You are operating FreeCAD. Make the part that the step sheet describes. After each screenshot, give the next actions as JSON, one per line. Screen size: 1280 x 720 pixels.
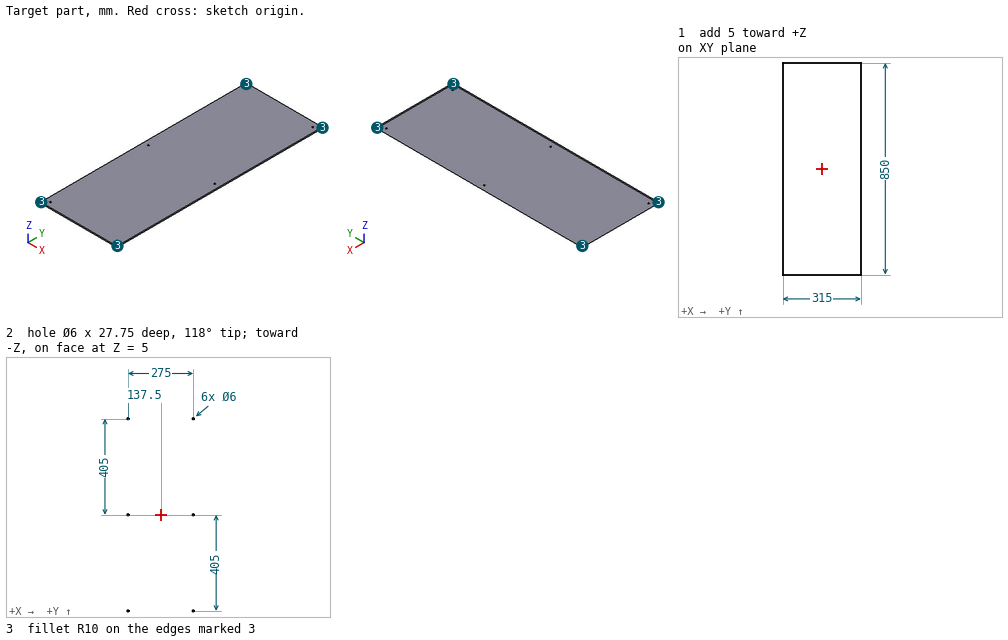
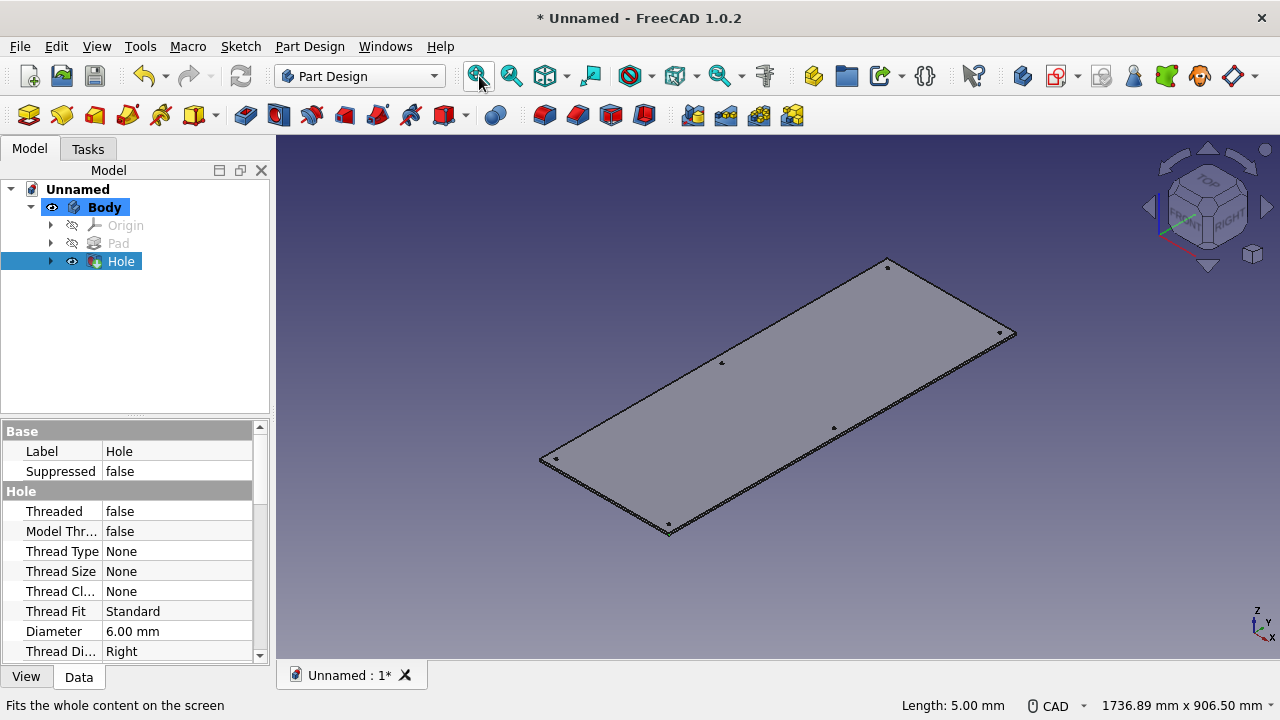
{"action": "scroll", "coordinate": [540, 459], "scroll_direction": "up", "scroll_amount": 14}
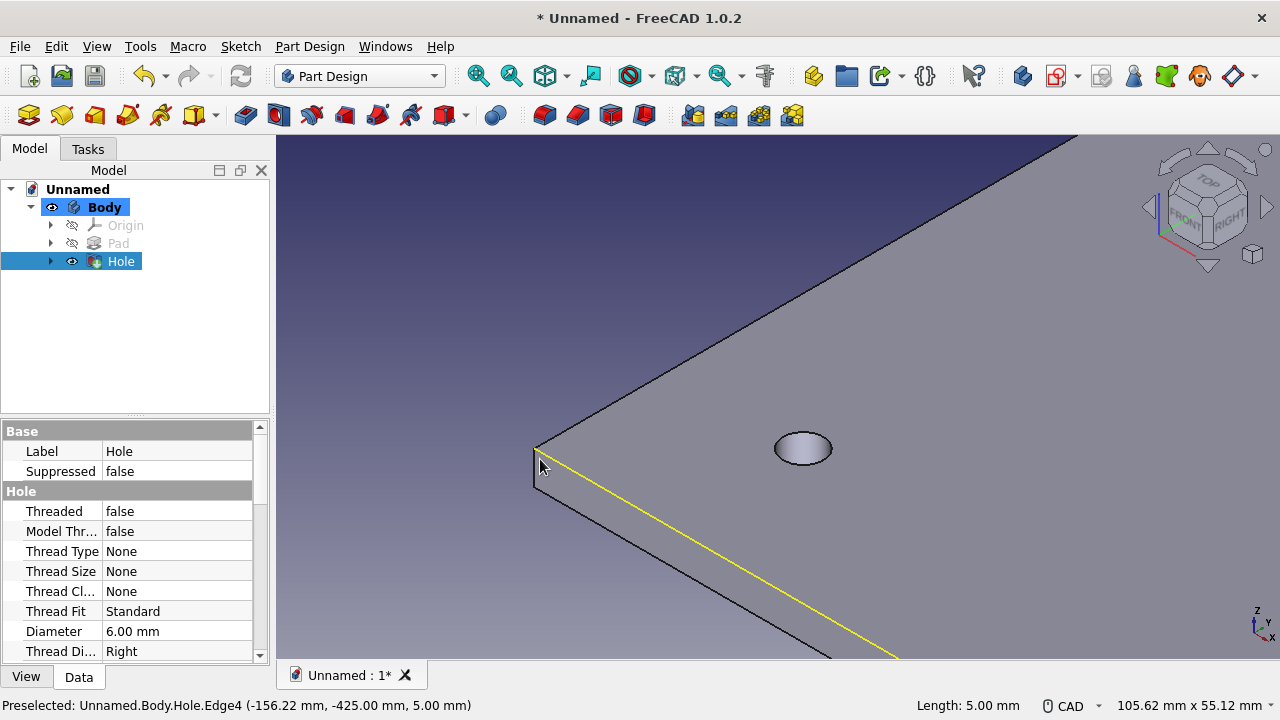
{"action": "key", "text": "v f"}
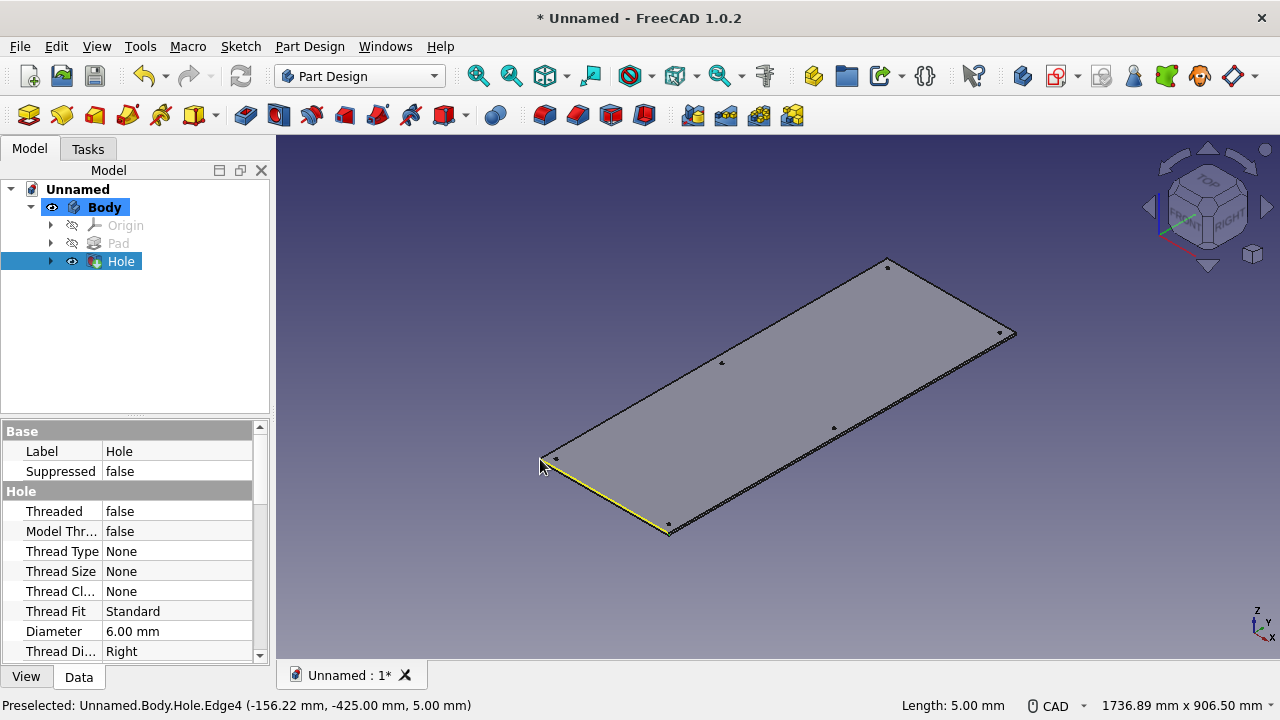
{"action": "key", "text": "2"}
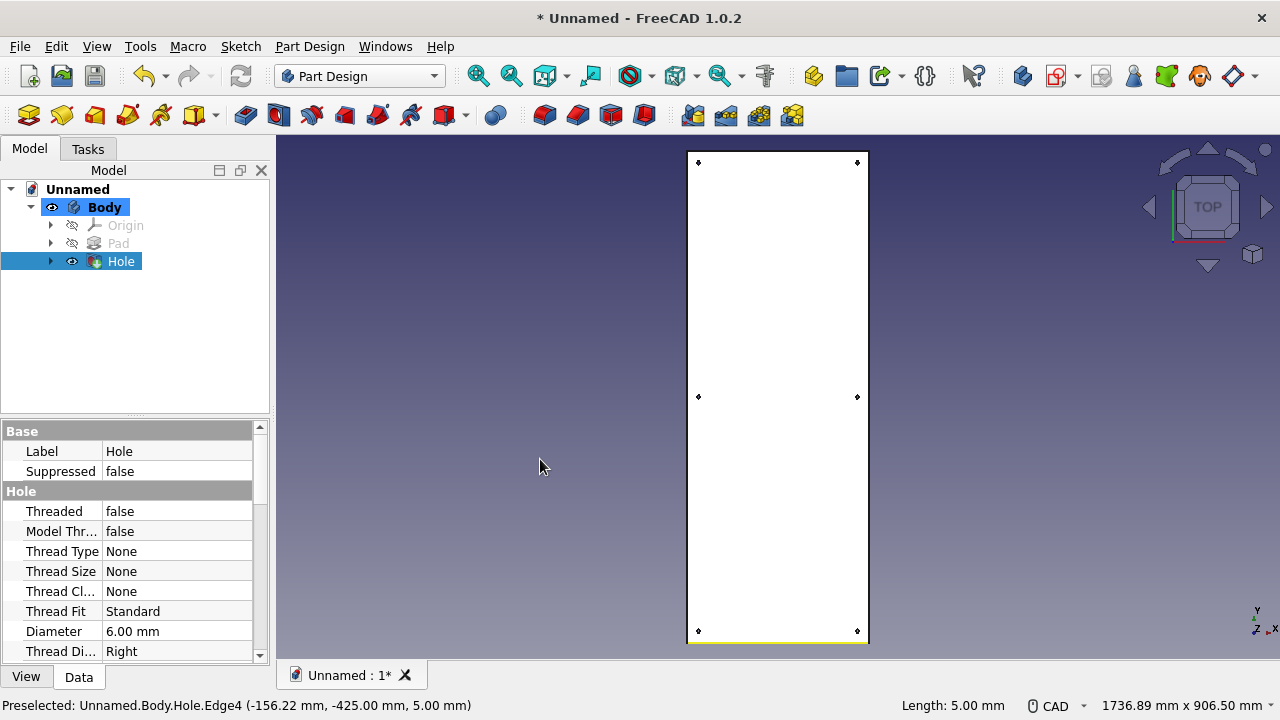
{"action": "key", "text": "1"}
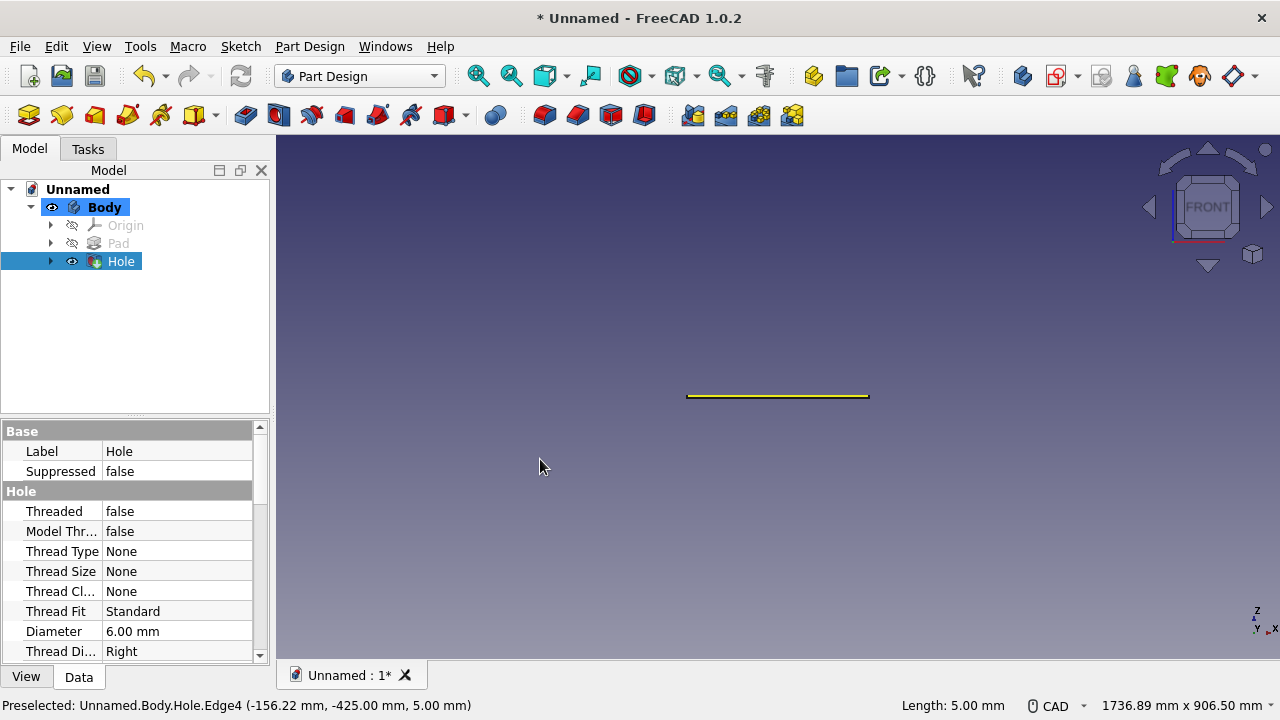
{"action": "key", "text": "v f"}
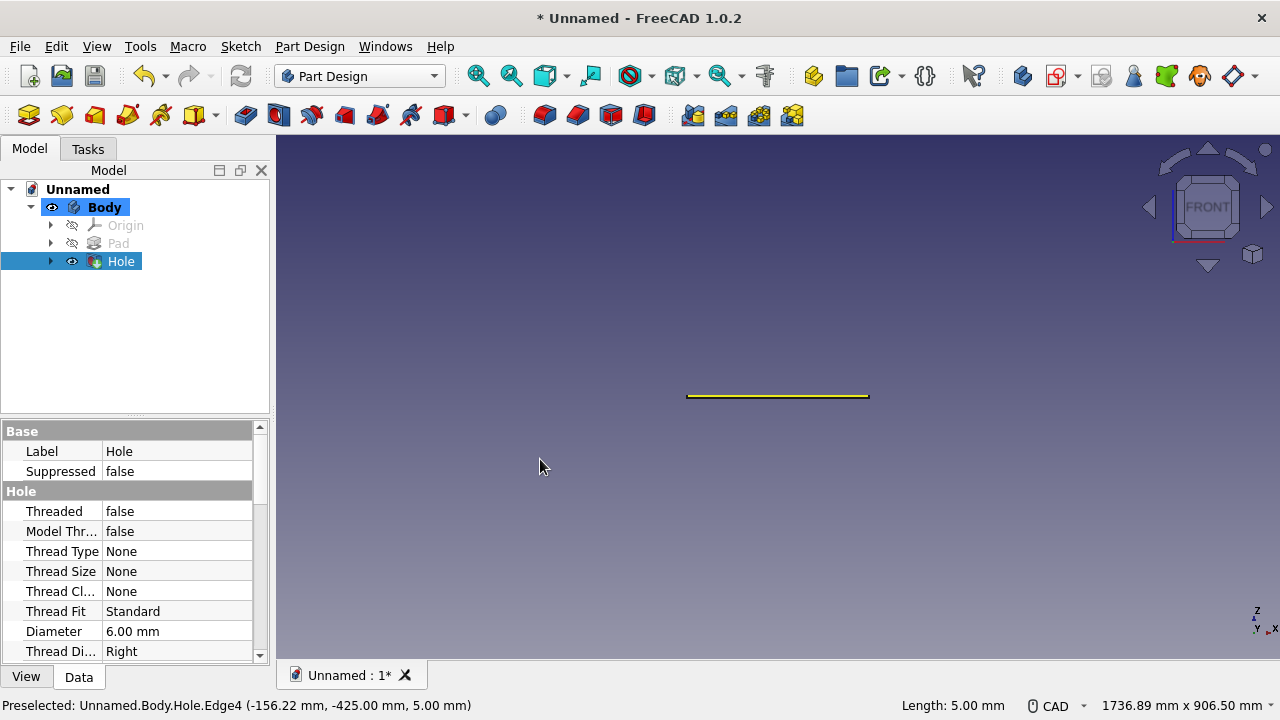
{"action": "scroll", "coordinate": [687, 396], "scroll_direction": "up", "scroll_amount": 14}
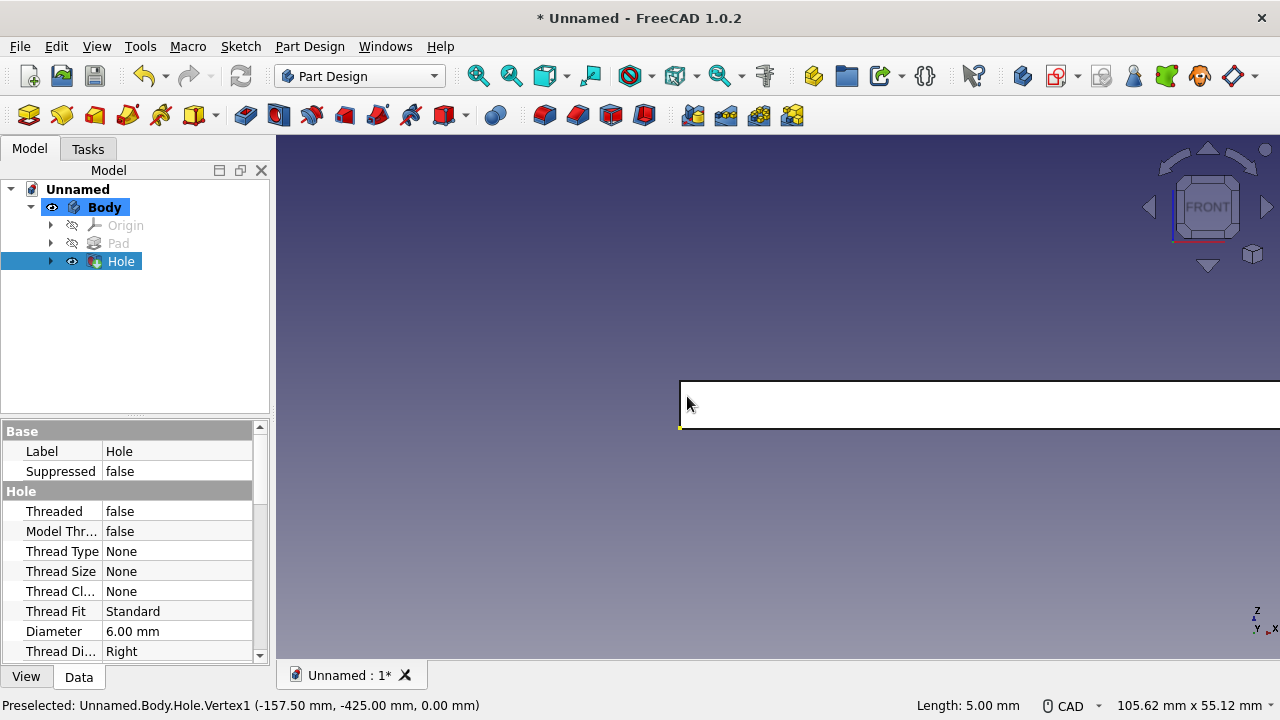
{"action": "left_click", "coordinate": [680, 404], "text": "ctrl"}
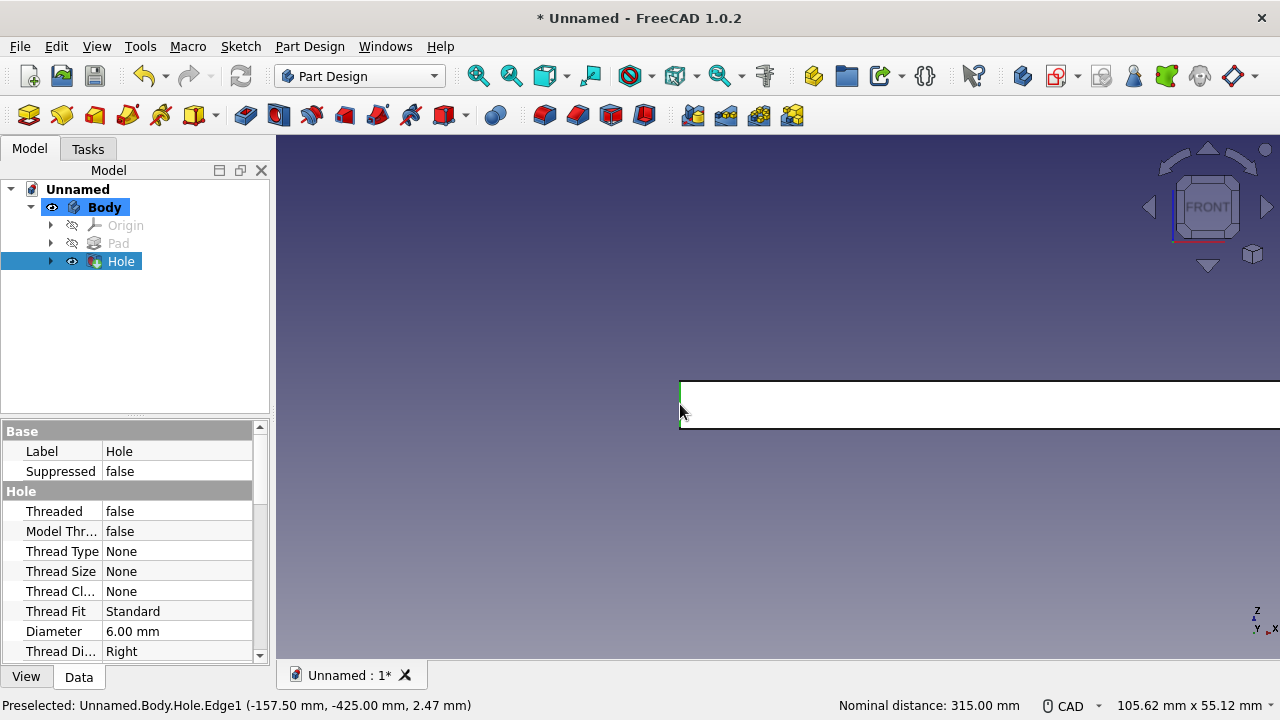
{"action": "key", "text": "v f"}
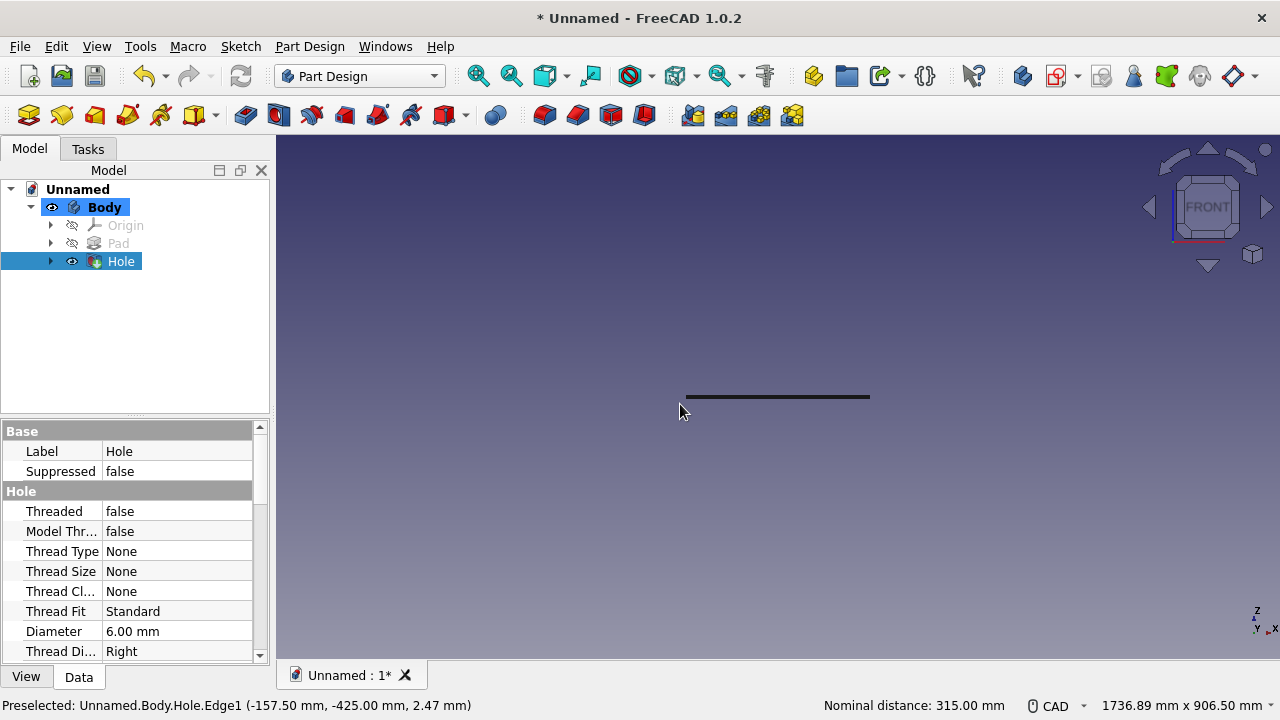
{"action": "key", "text": "3"}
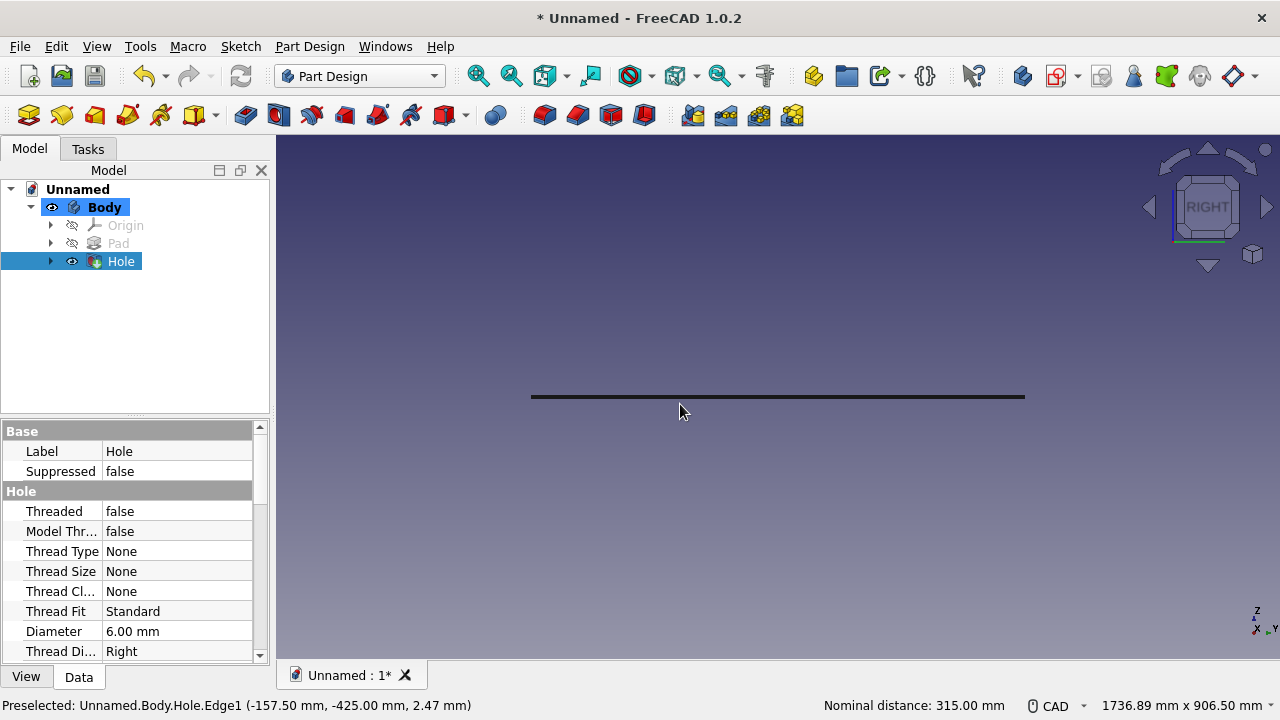
{"action": "scroll", "coordinate": [1024, 396], "scroll_direction": "up", "scroll_amount": 14}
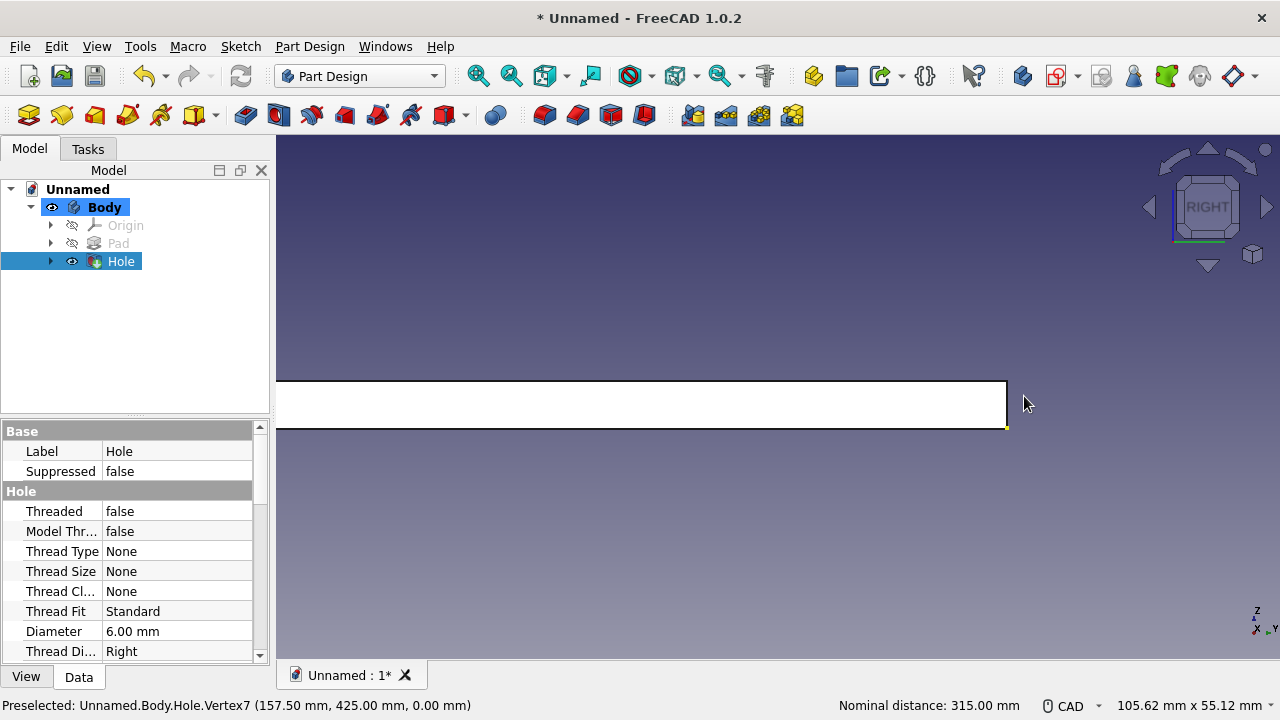
{"action": "left_click", "coordinate": [1007, 404], "text": "ctrl"}